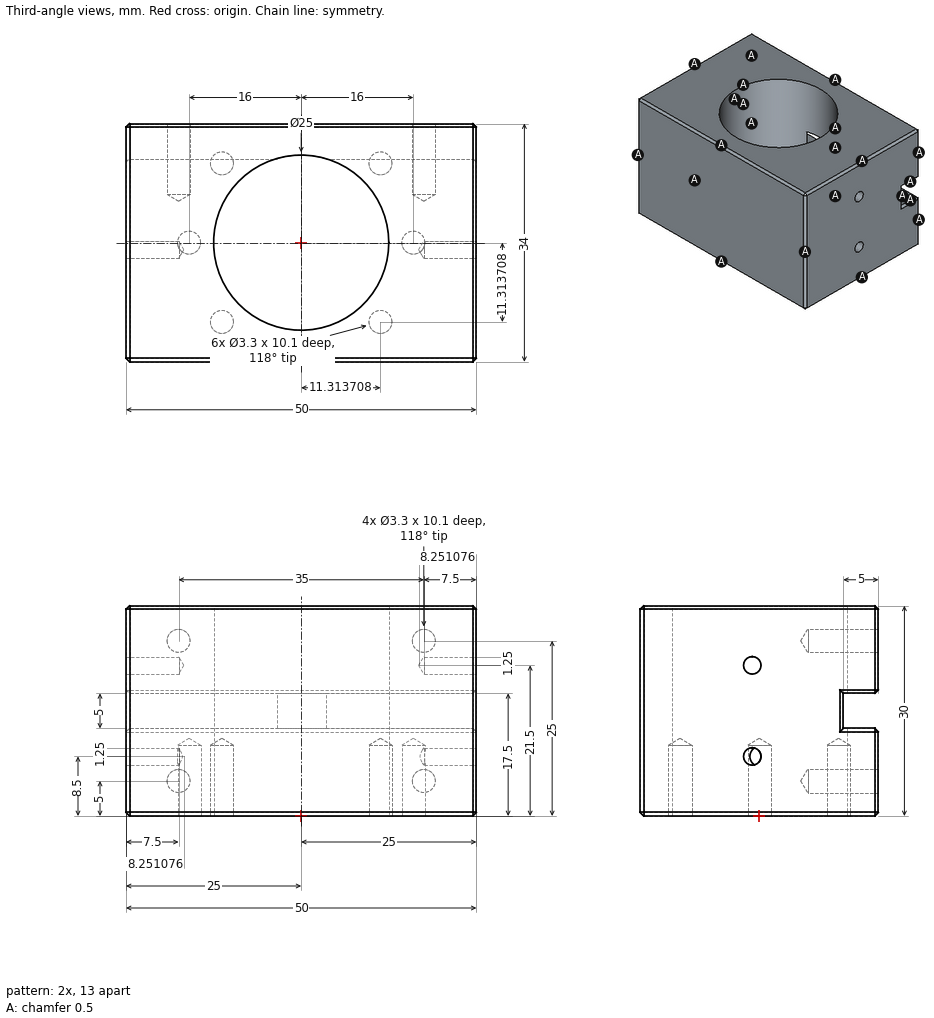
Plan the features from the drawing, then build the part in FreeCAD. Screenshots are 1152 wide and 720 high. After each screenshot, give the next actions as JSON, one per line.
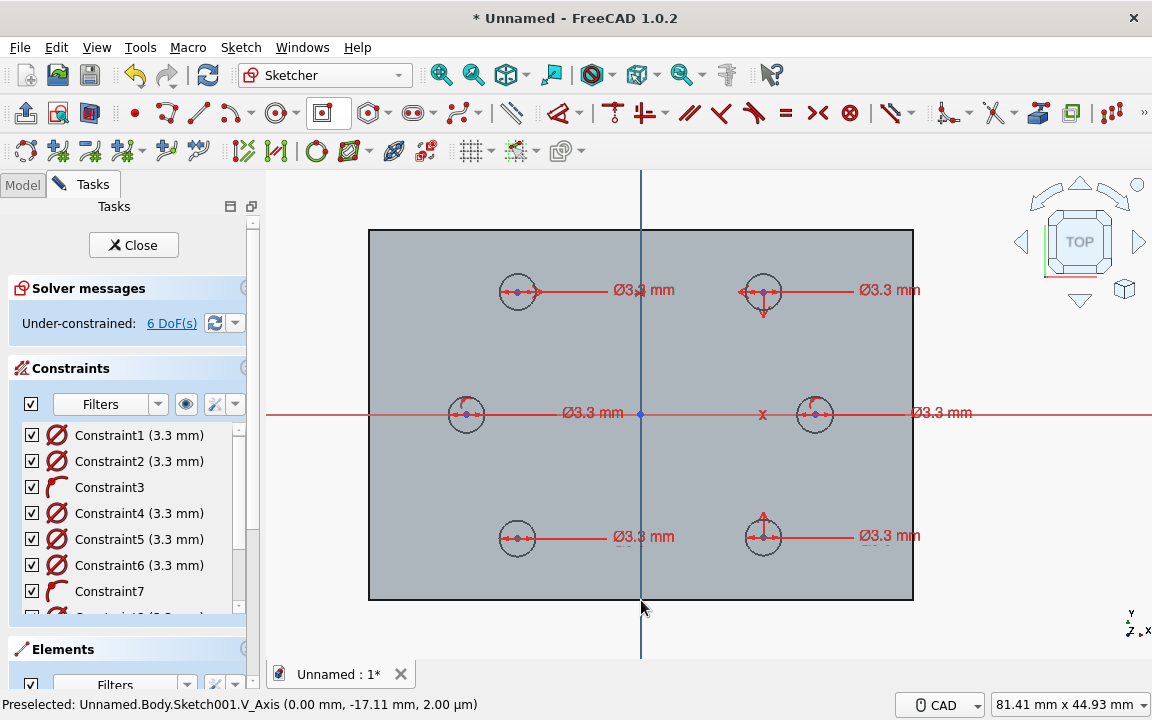
{"action": "key", "text": "s"}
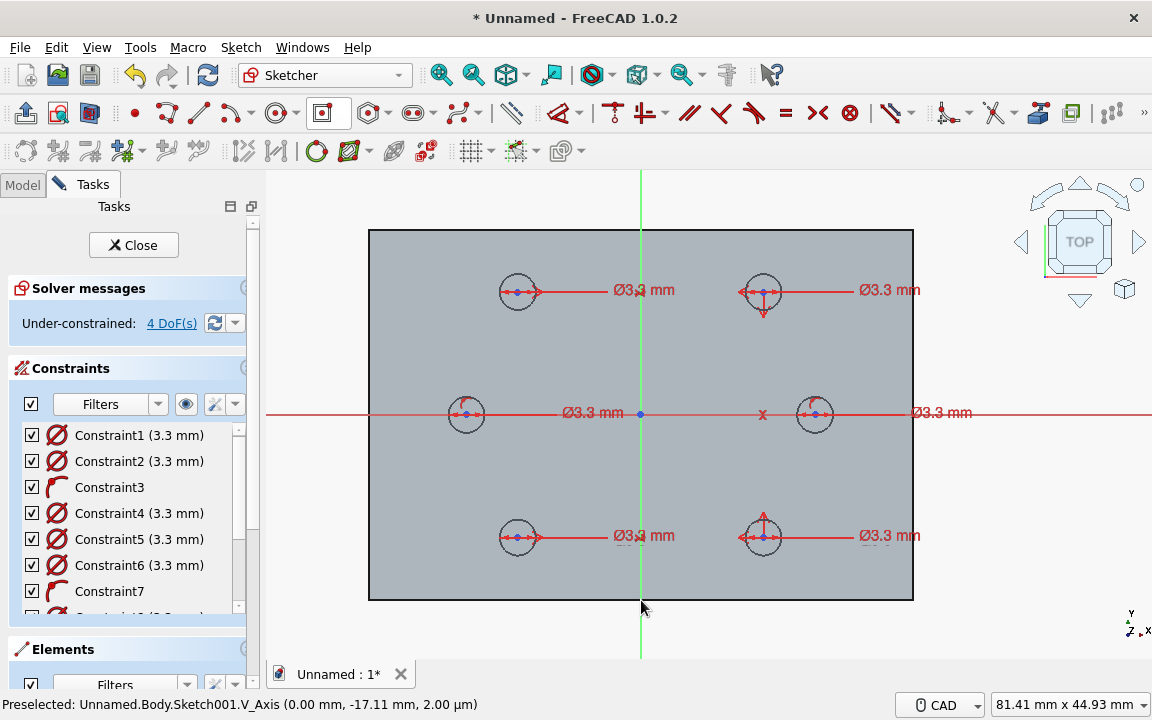
{"action": "key", "text": "d"}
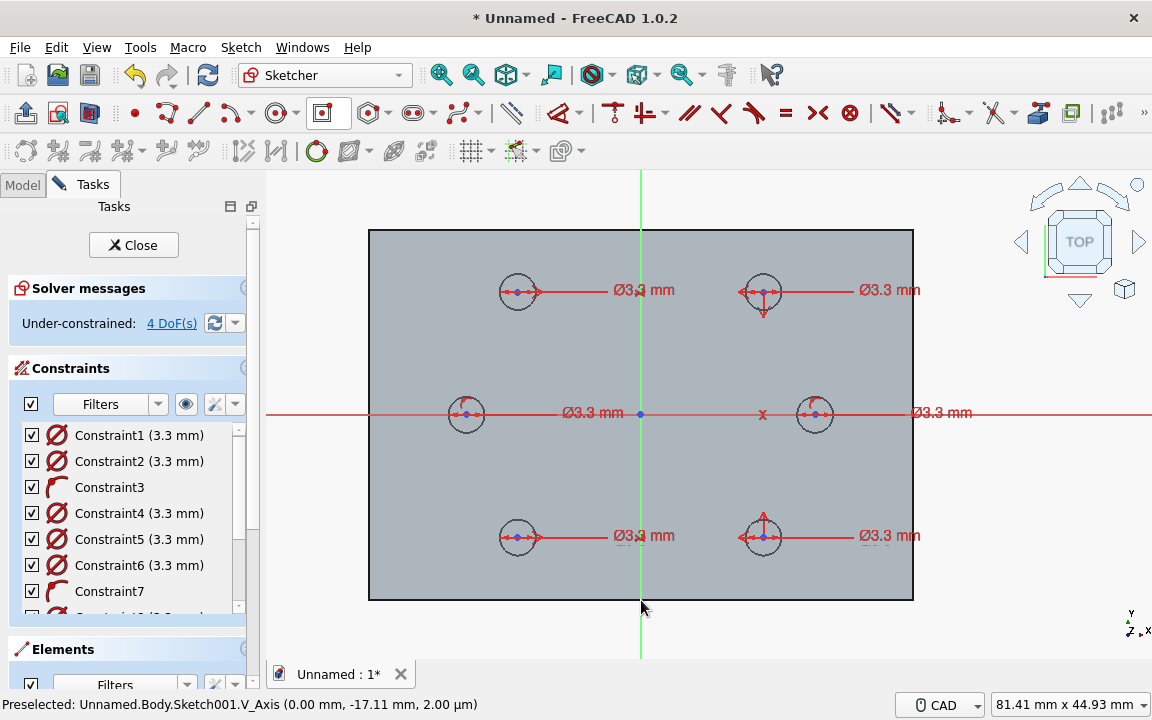
{"action": "left_click", "coordinate": [815, 415]}
{"action": "left_click", "coordinate": [728, 449]}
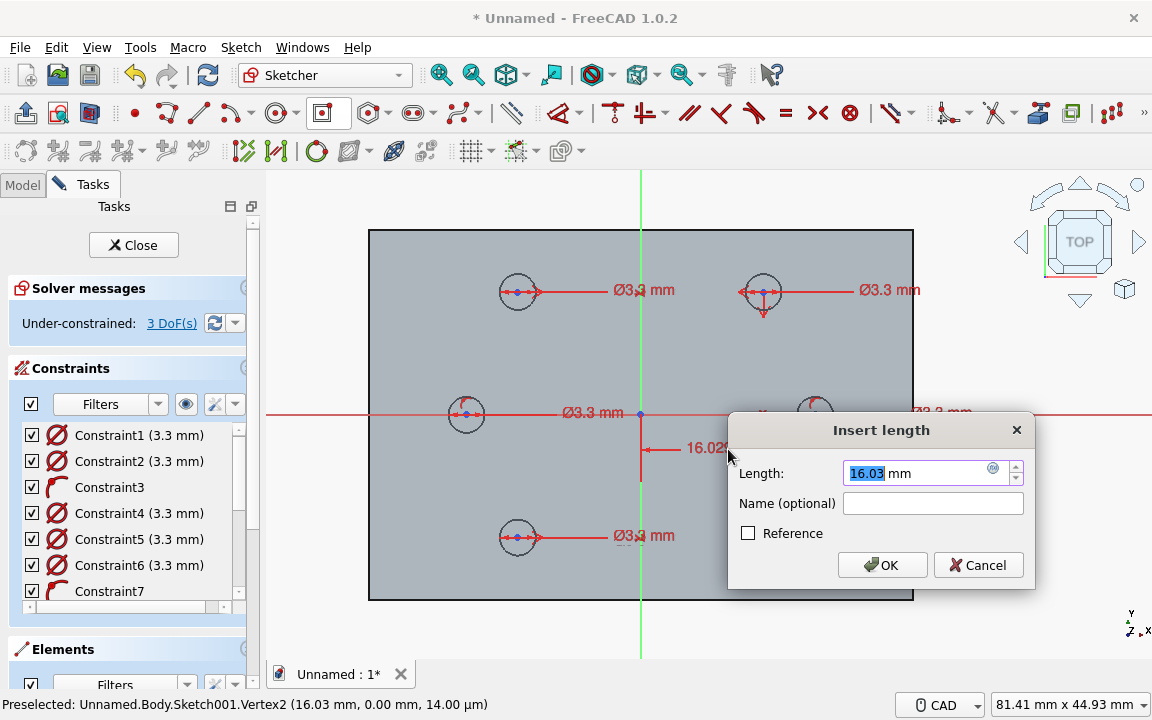
{"action": "type", "text": "16"}
{"action": "key", "text": "Return"}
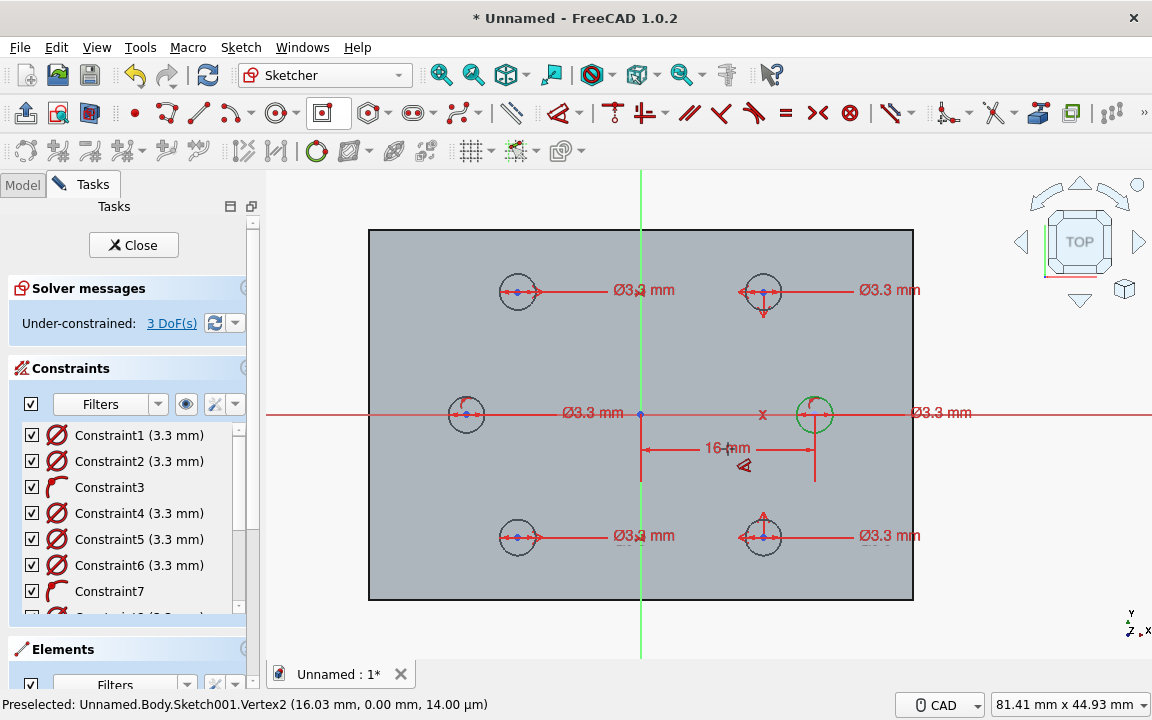
{"action": "left_click", "coordinate": [467, 415]}
{"action": "left_click", "coordinate": [554, 449]}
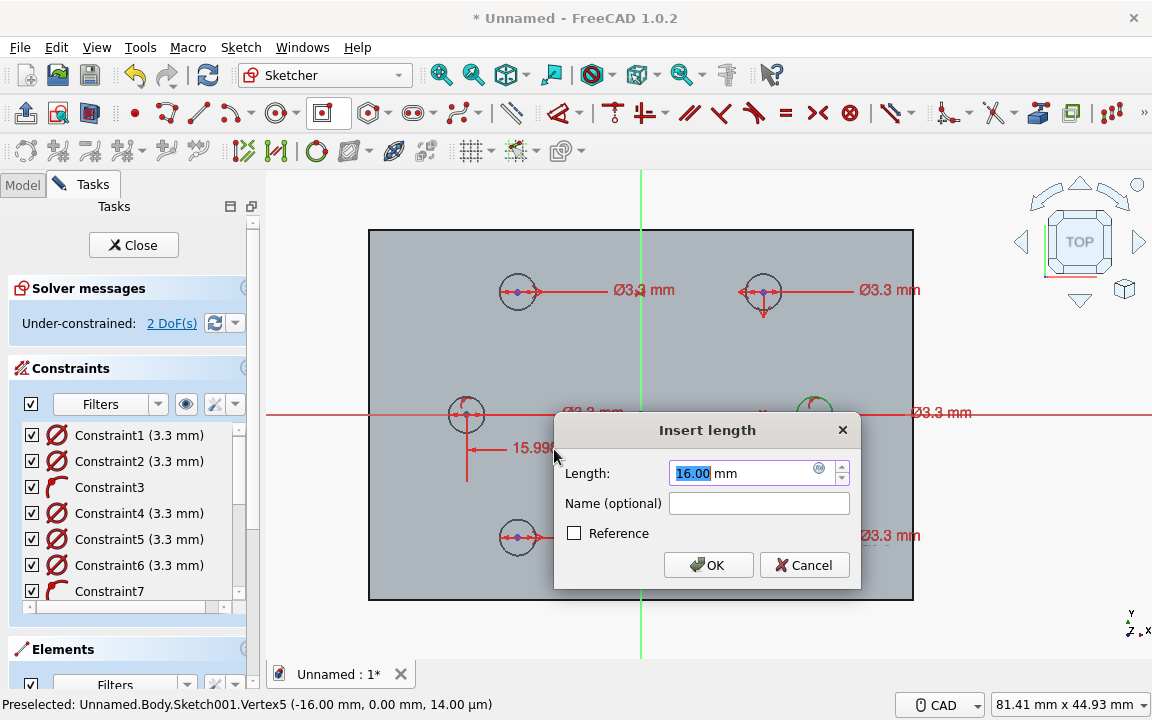
{"action": "type", "text": "16"}
{"action": "key", "text": "Return"}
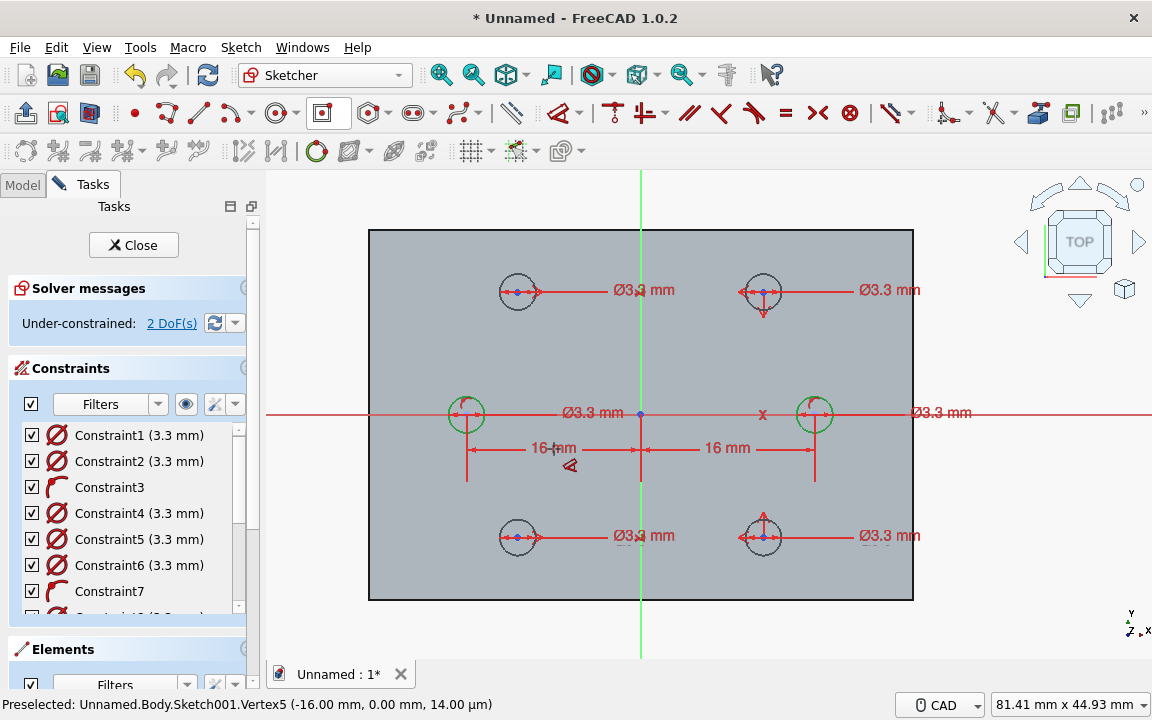
{"action": "left_click", "coordinate": [764, 538]}
{"action": "left_click", "coordinate": [702, 572]}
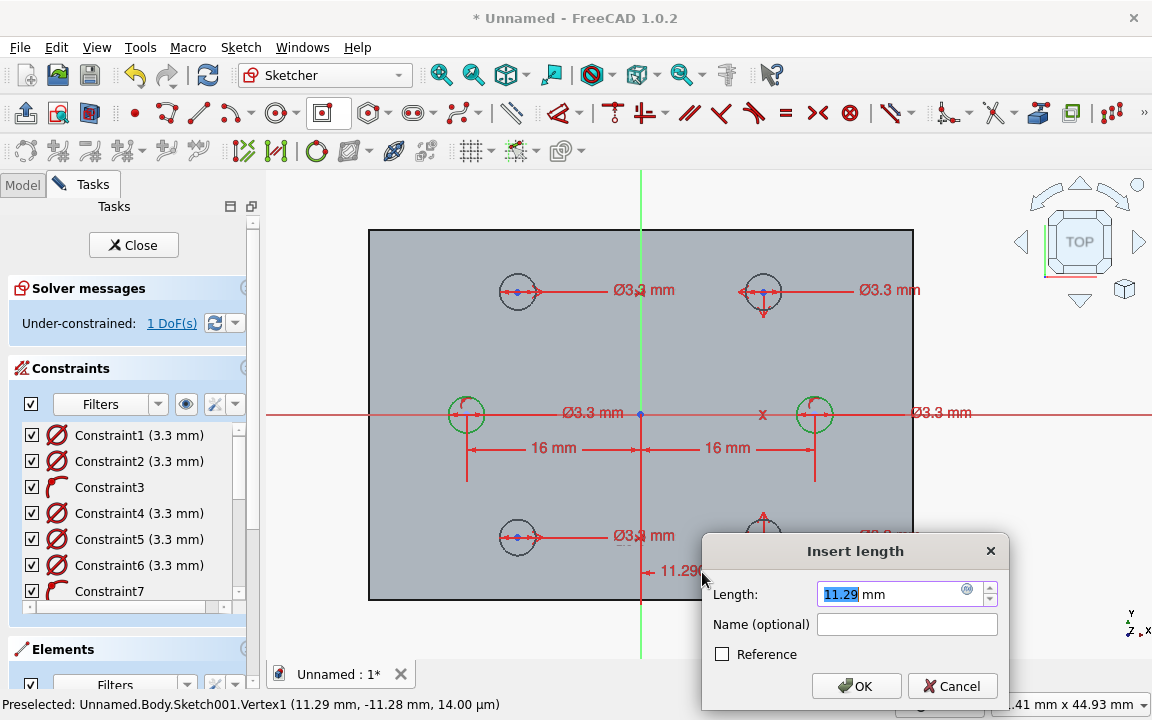
{"action": "type", "text": "11.313708"}
{"action": "key", "text": "Return"}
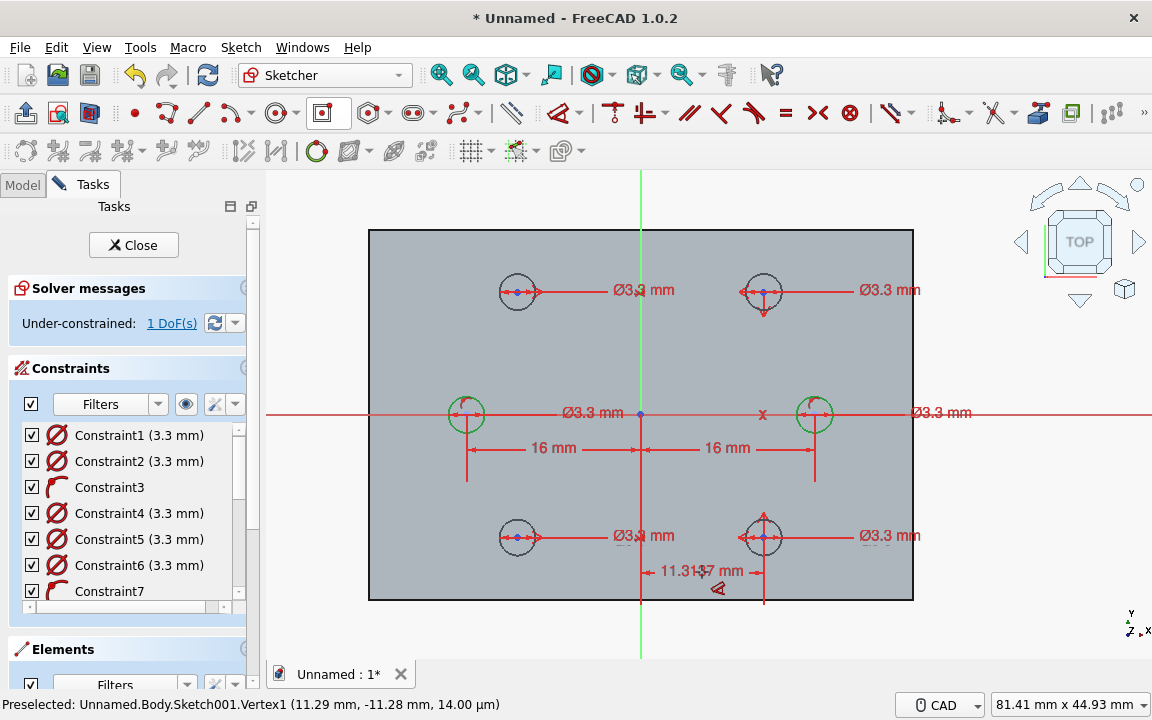
{"action": "left_click", "coordinate": [764, 538]}
{"action": "left_click", "coordinate": [798, 476]}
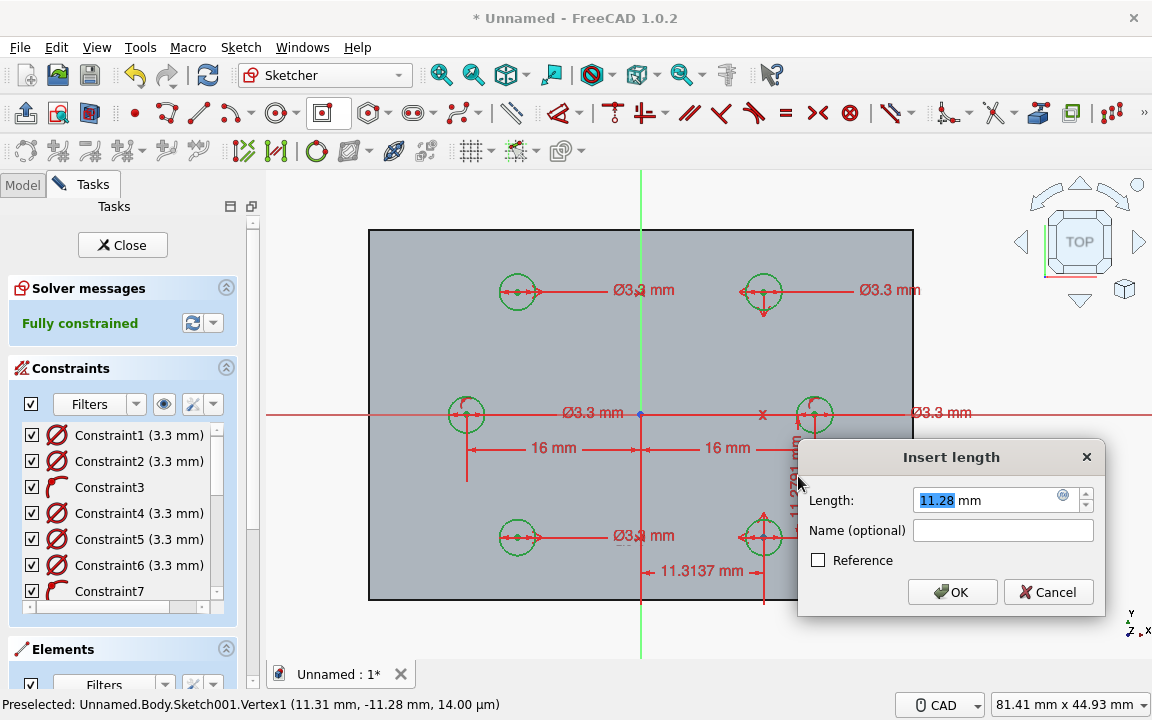
{"action": "type", "text": "11.313708"}
{"action": "key", "text": "Return"}
{"action": "key", "text": "Escape"}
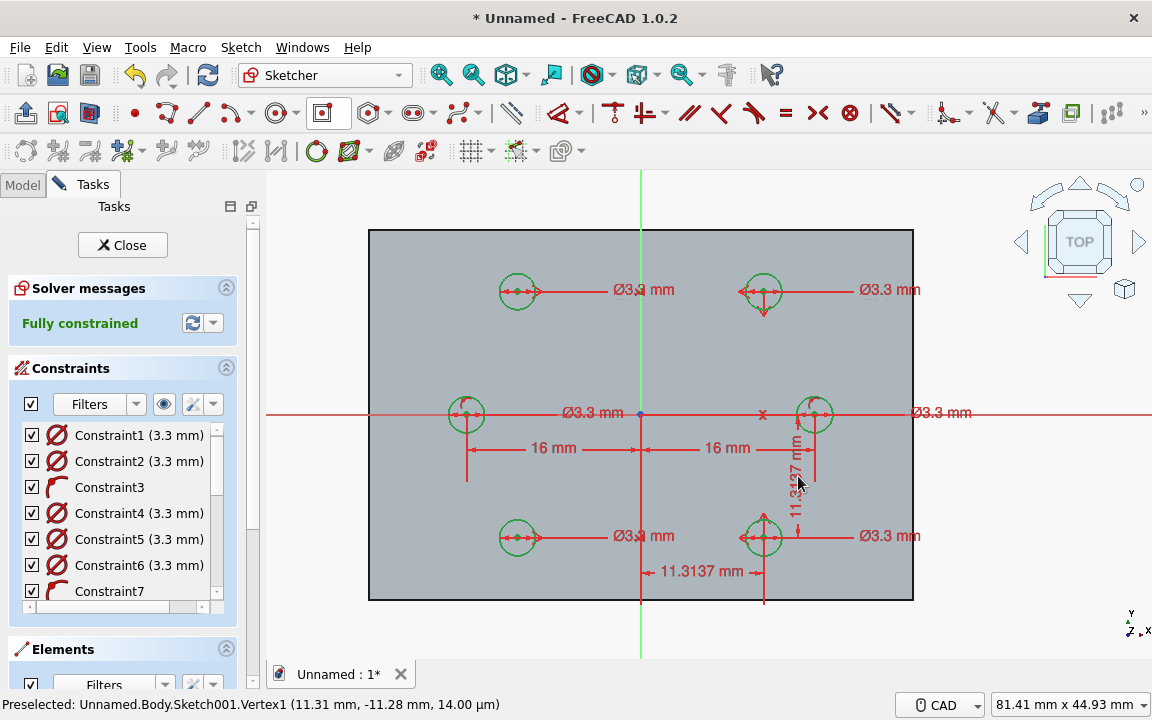
{"action": "left_click", "coordinate": [123, 245]}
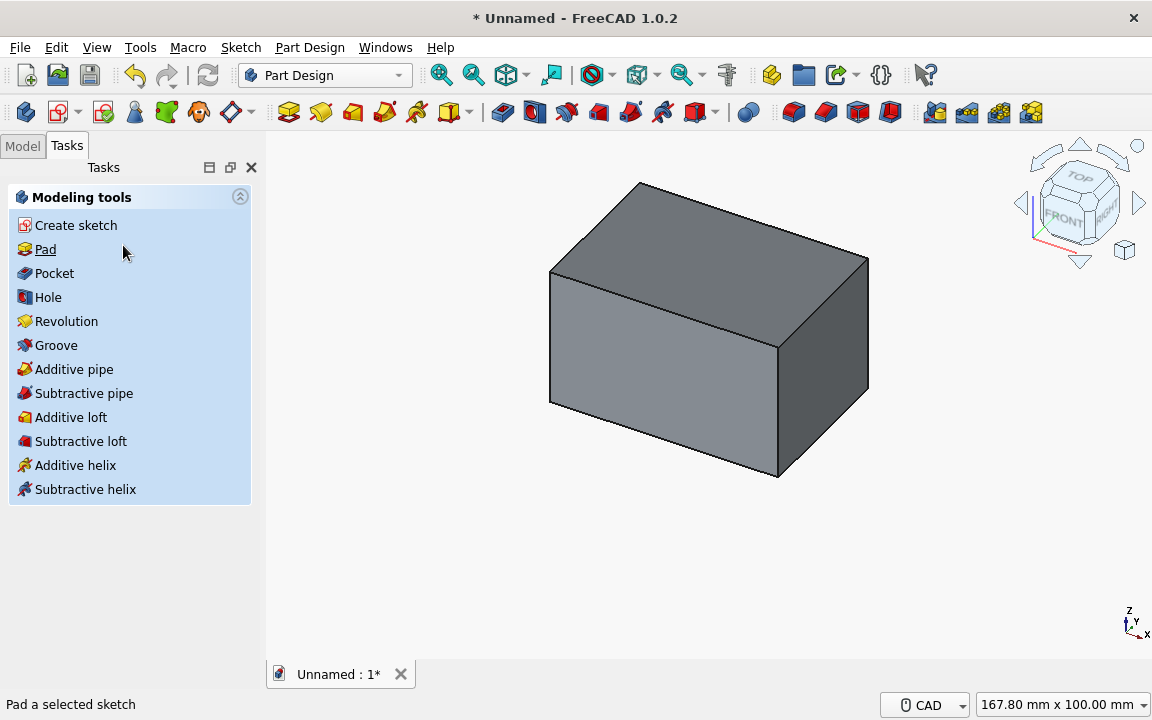
{"action": "left_click", "coordinate": [536, 112]}